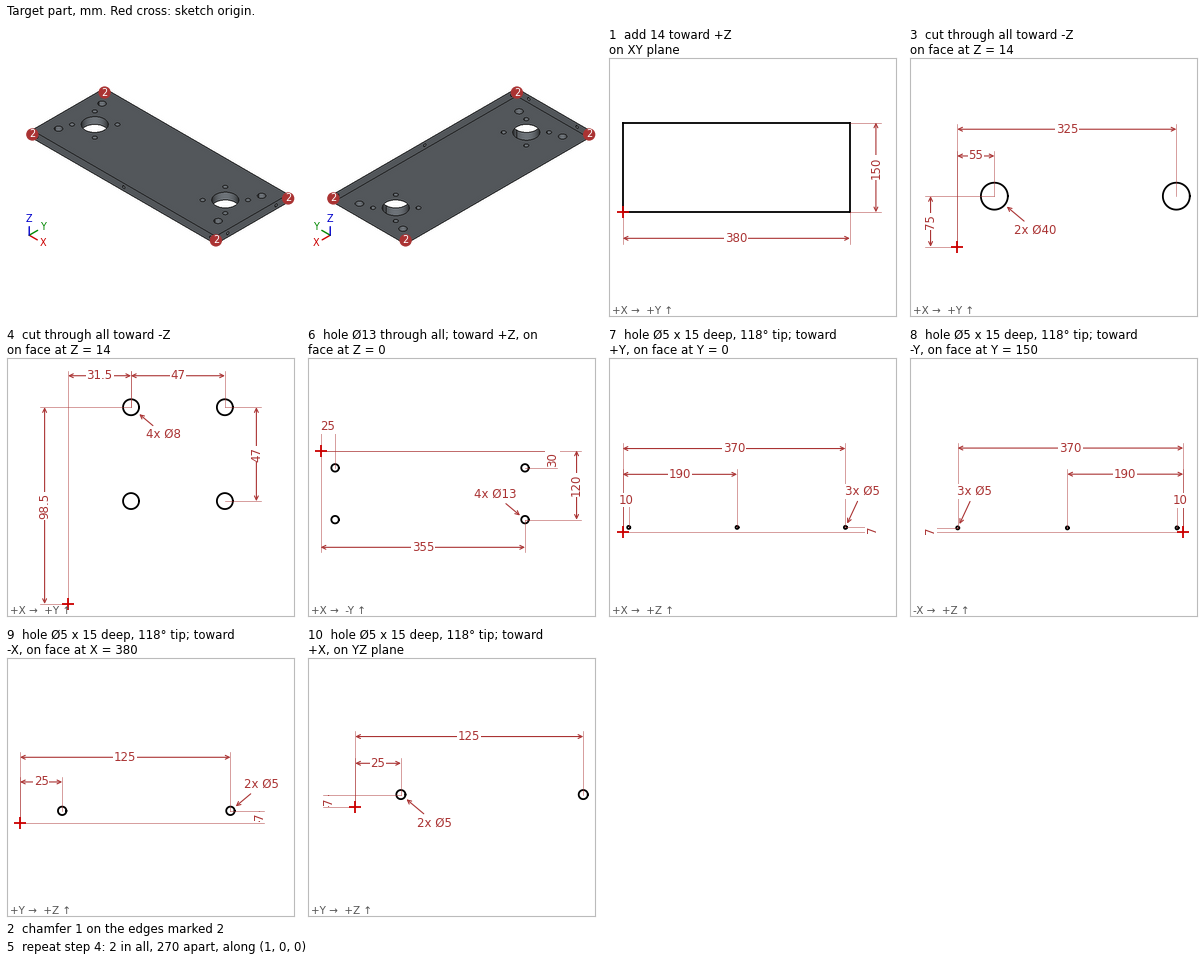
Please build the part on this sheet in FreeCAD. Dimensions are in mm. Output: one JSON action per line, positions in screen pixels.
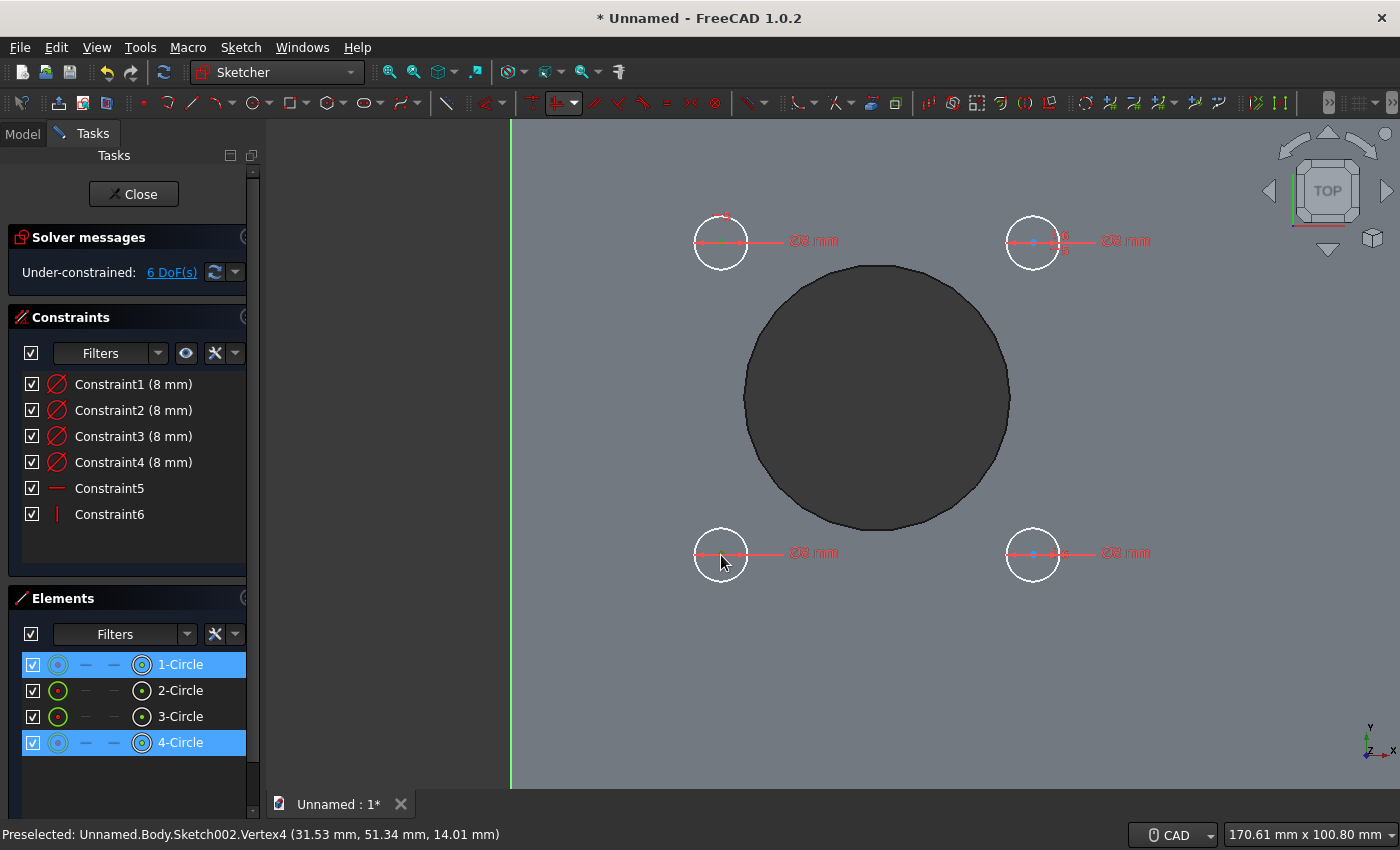
{"action": "left_click", "coordinate": [576, 104]}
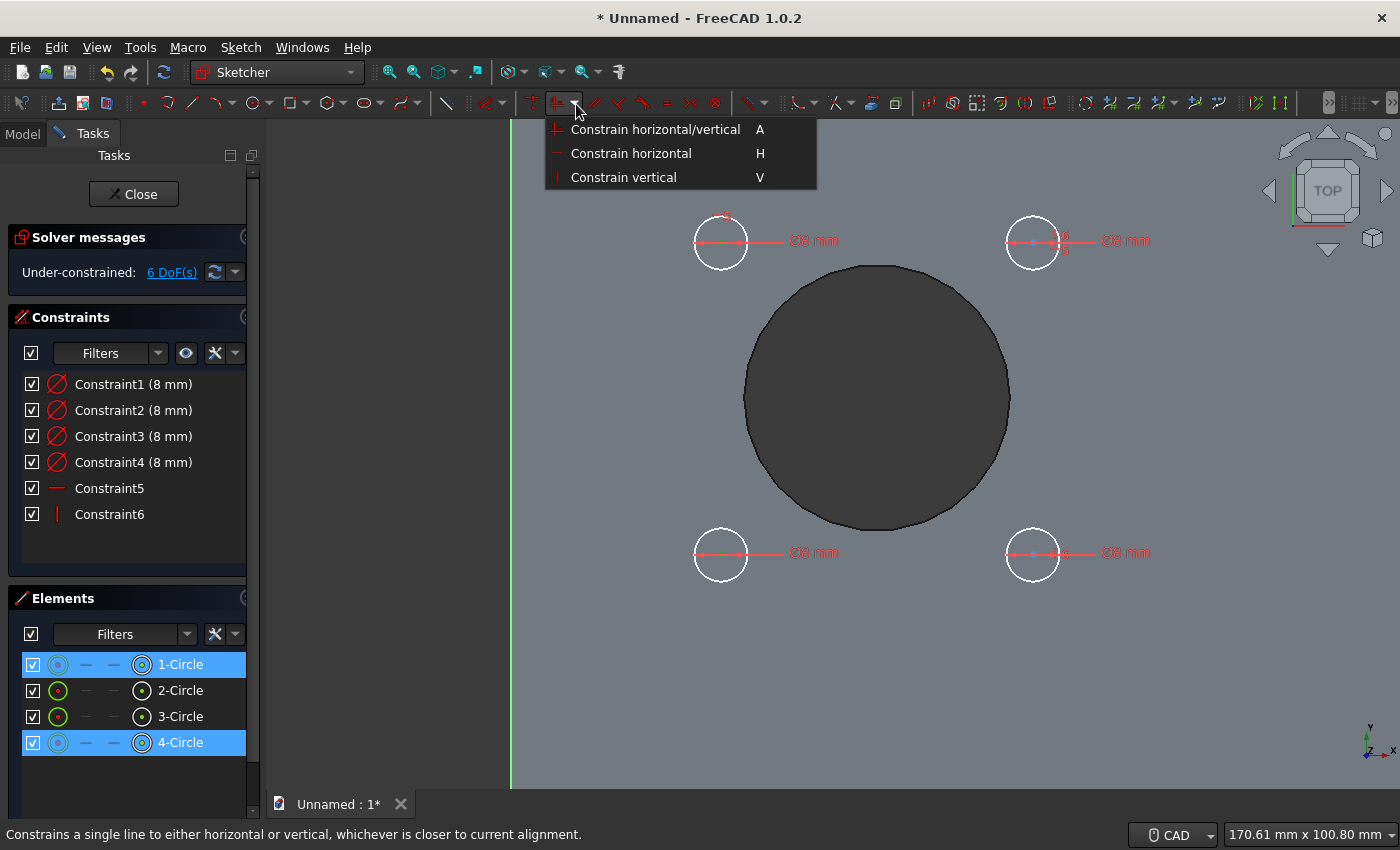
{"action": "left_click", "coordinate": [681, 177]}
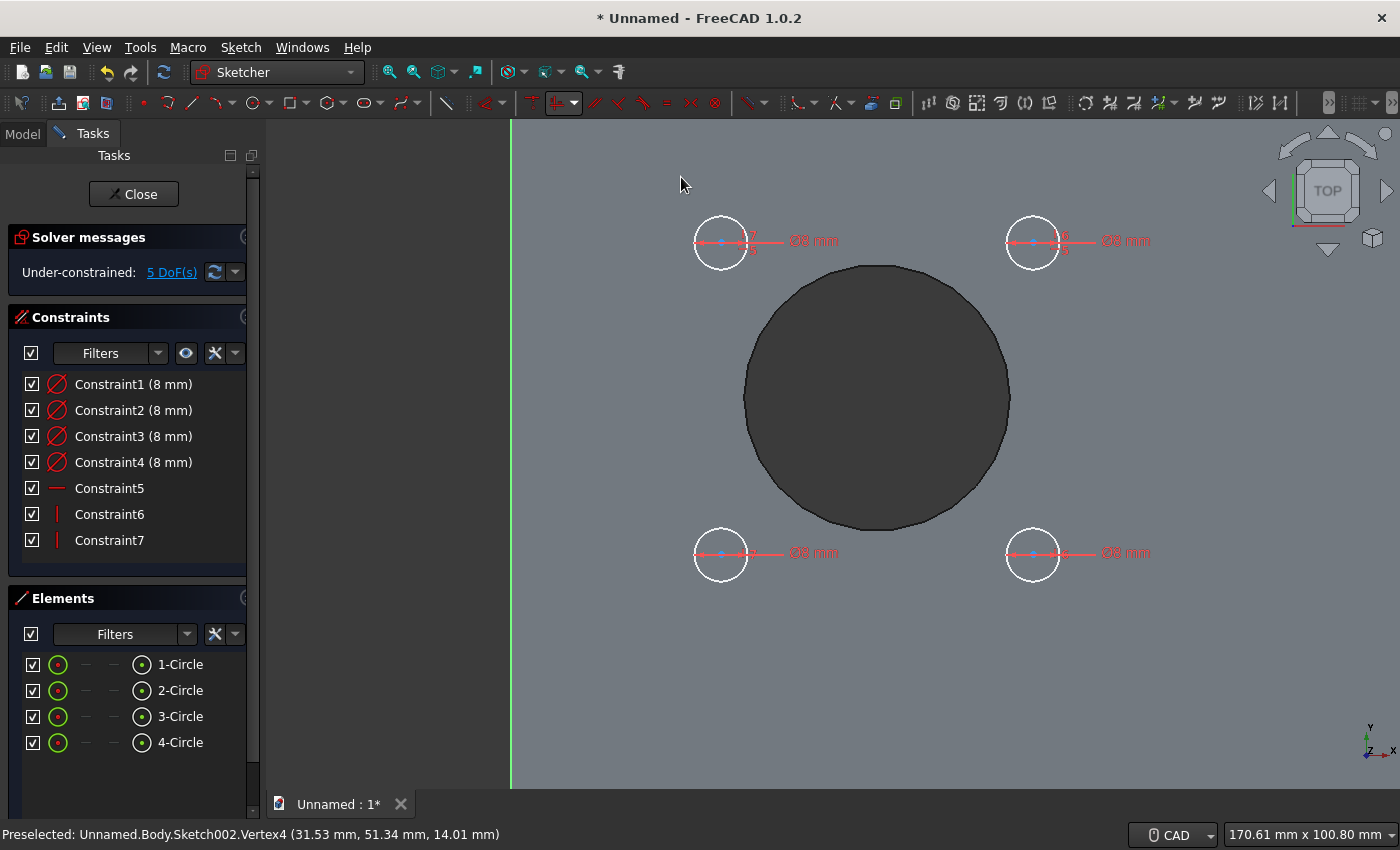
{"action": "left_click", "coordinate": [1033, 555]}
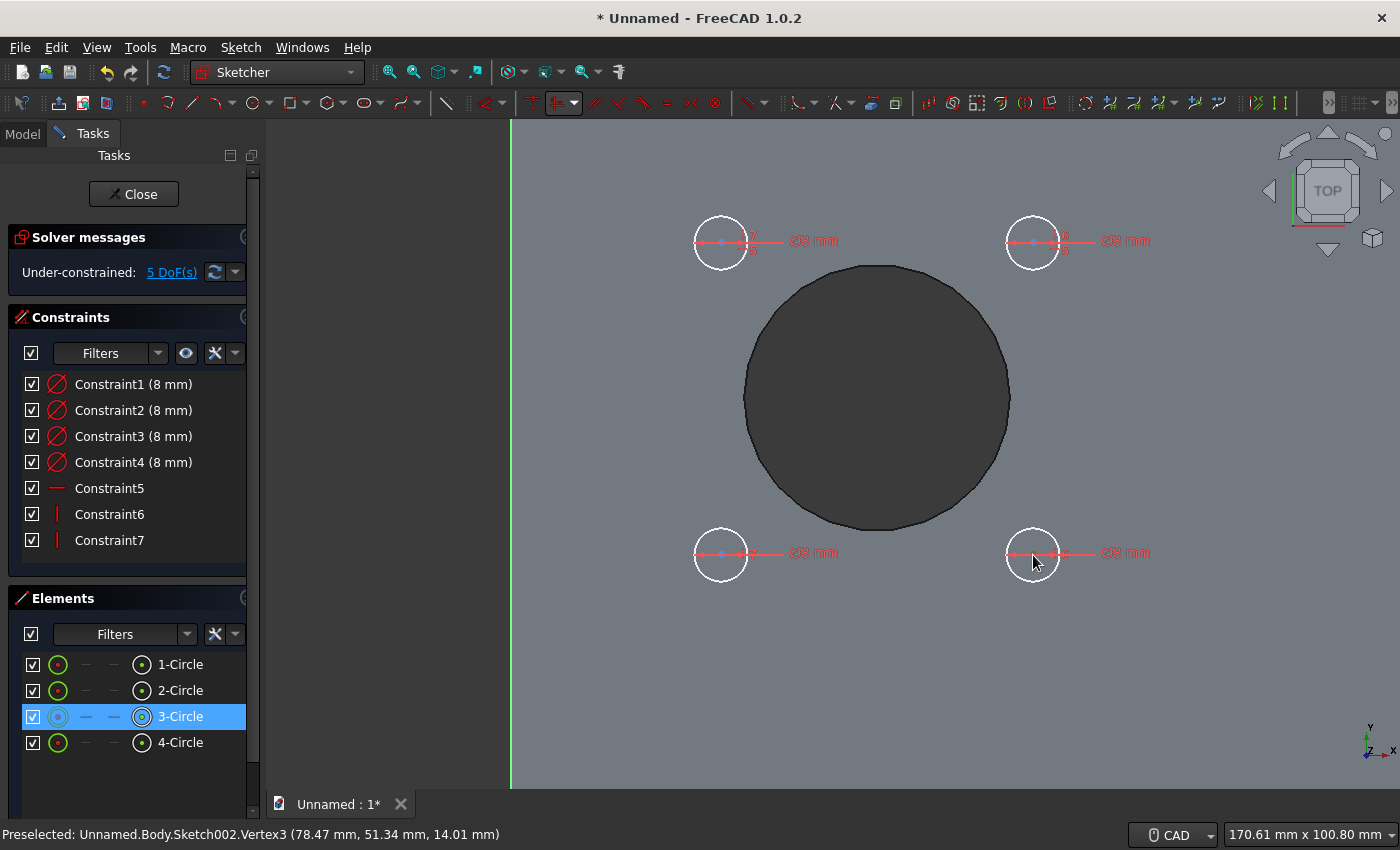
{"action": "left_click", "coordinate": [721, 555]}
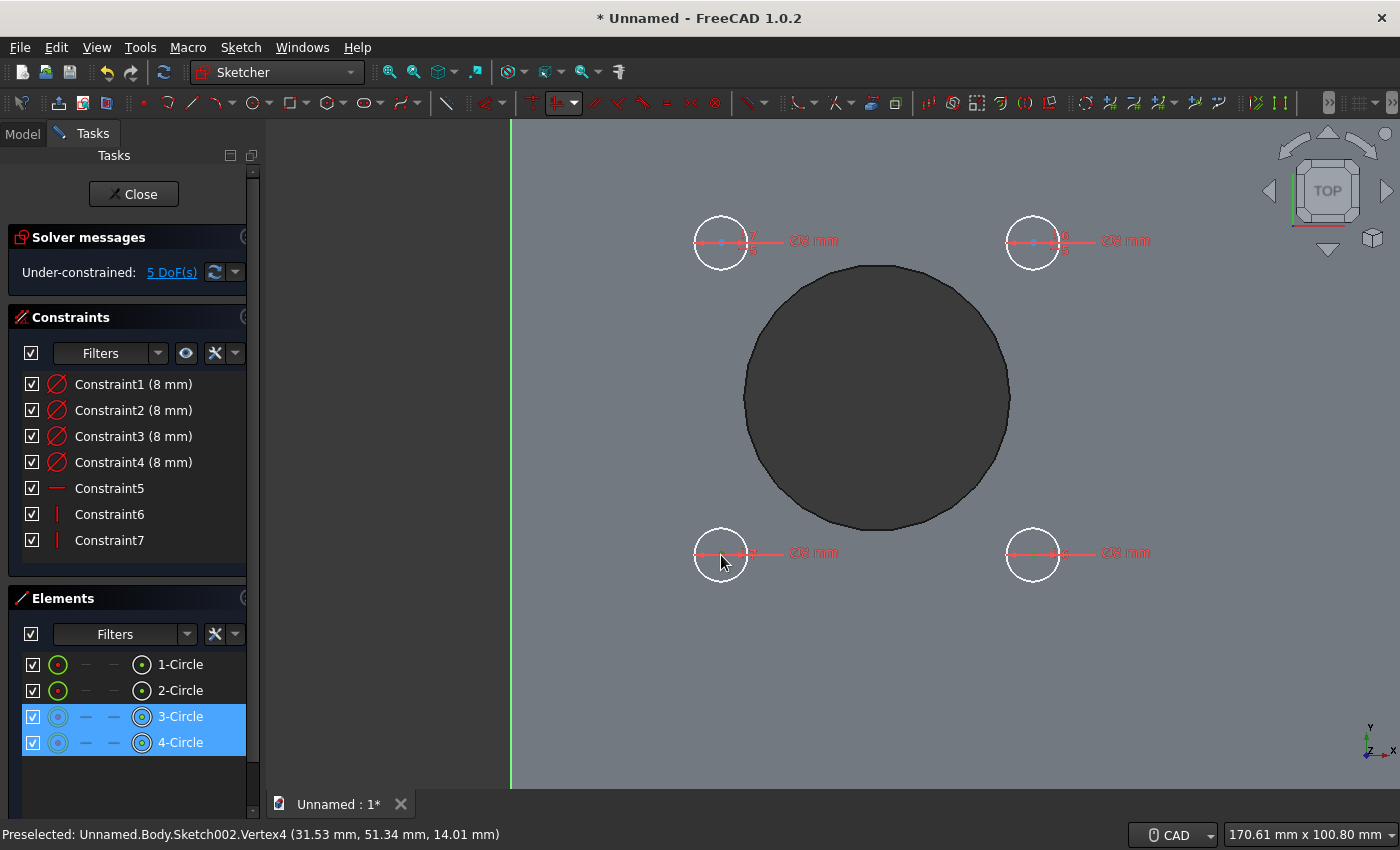
{"action": "key", "text": "h"}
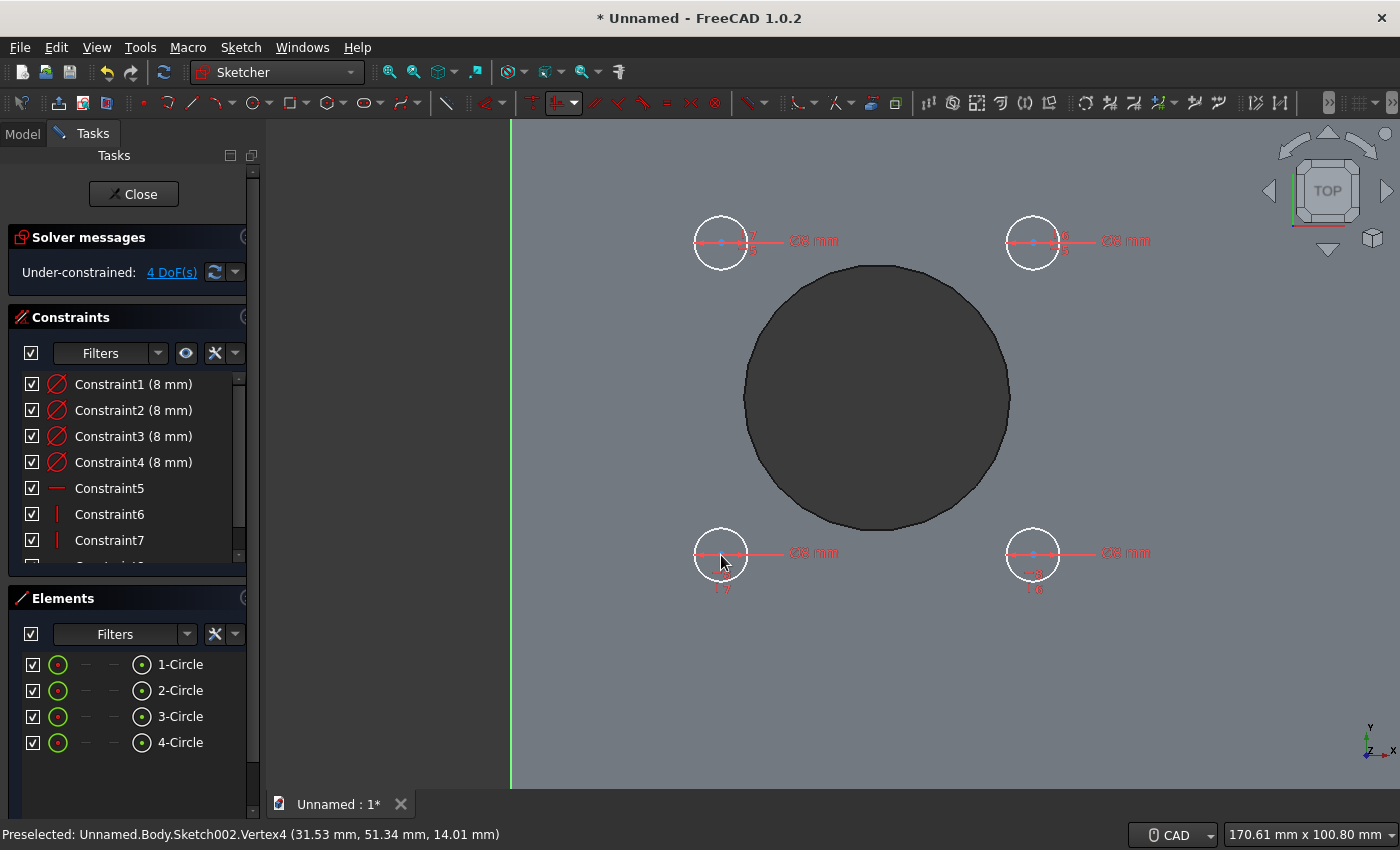
{"action": "key", "text": "d"}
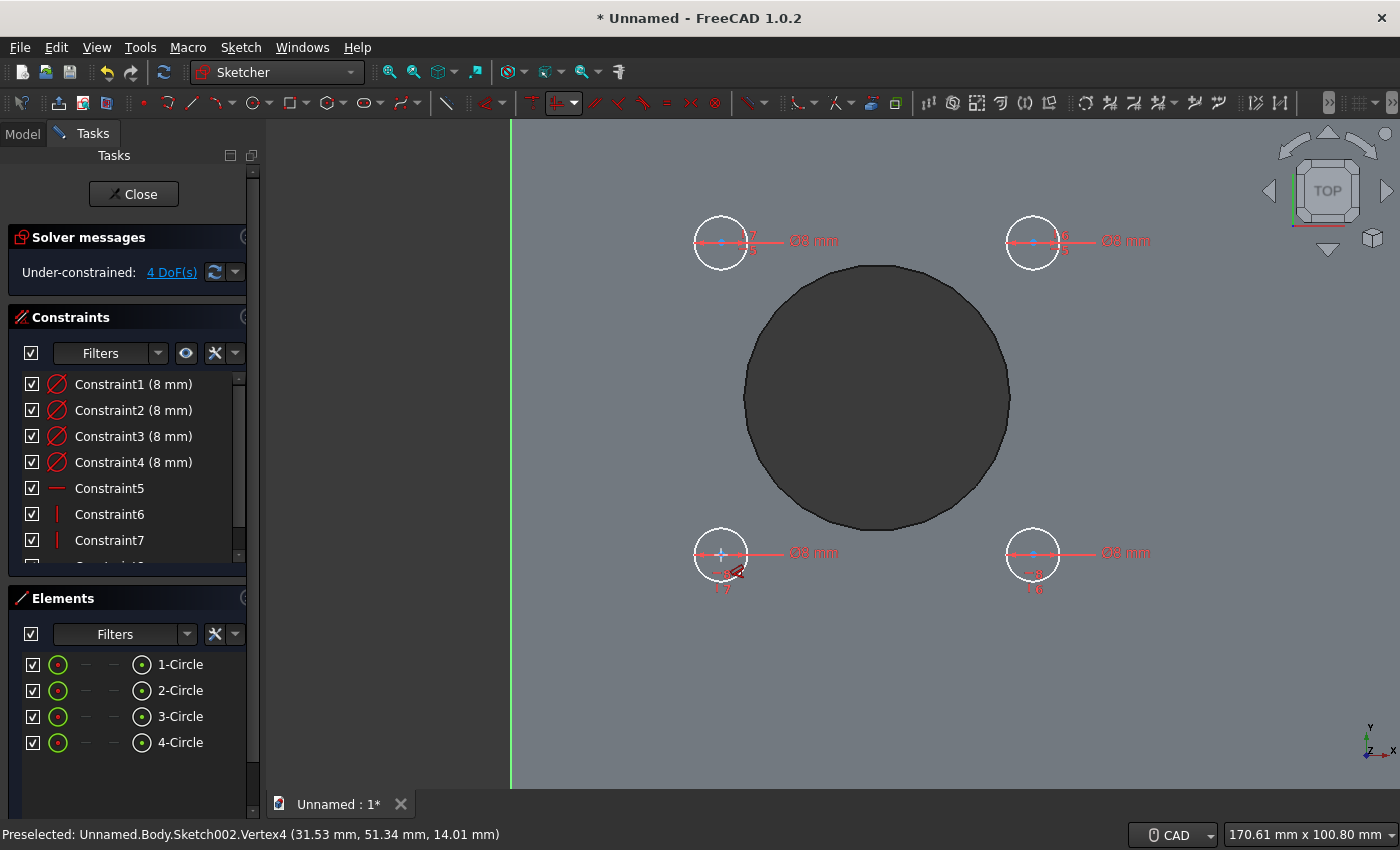
{"action": "left_click", "coordinate": [721, 243]}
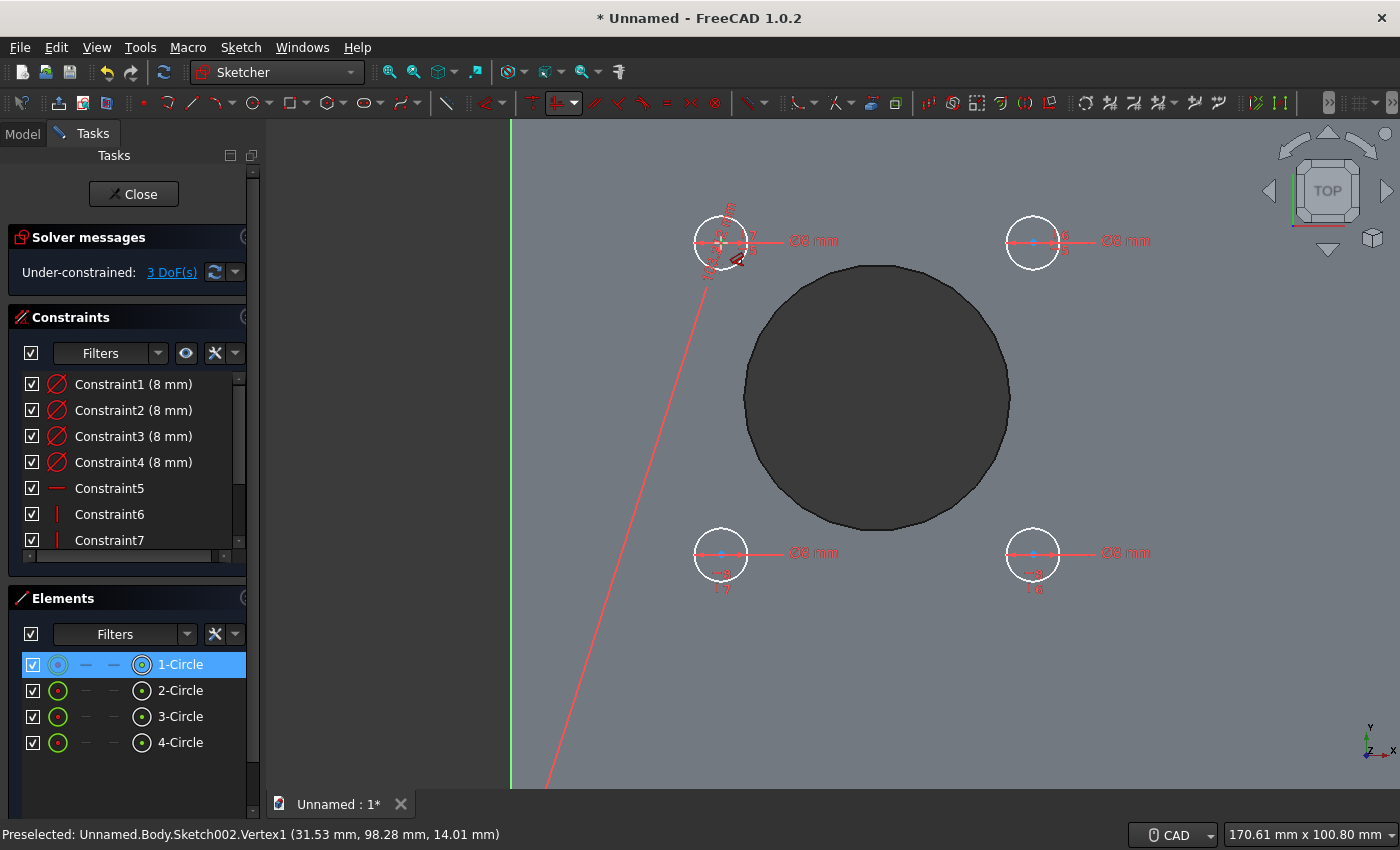
{"action": "left_click", "coordinate": [1033, 243]}
{"action": "left_click", "coordinate": [877, 209]}